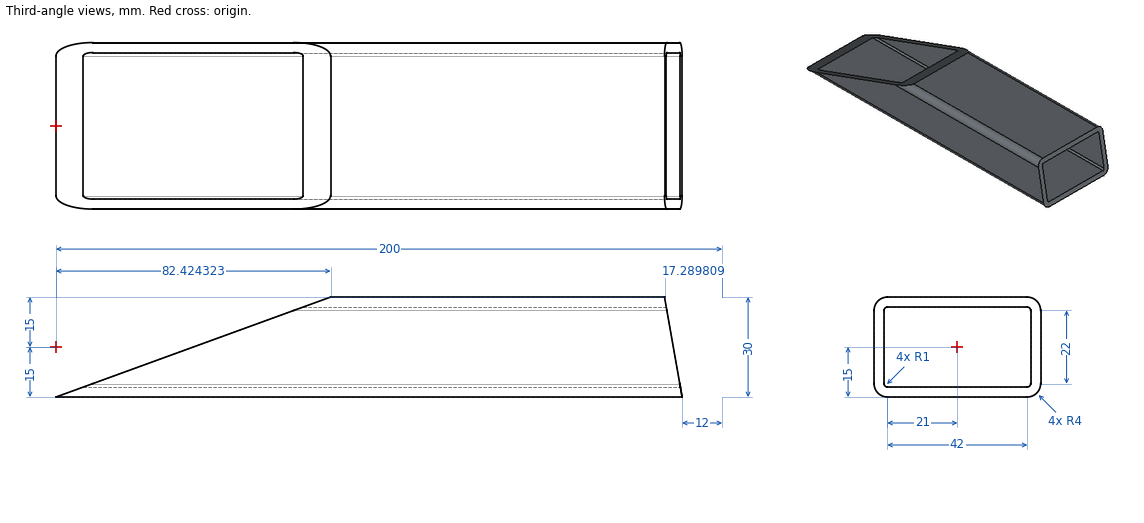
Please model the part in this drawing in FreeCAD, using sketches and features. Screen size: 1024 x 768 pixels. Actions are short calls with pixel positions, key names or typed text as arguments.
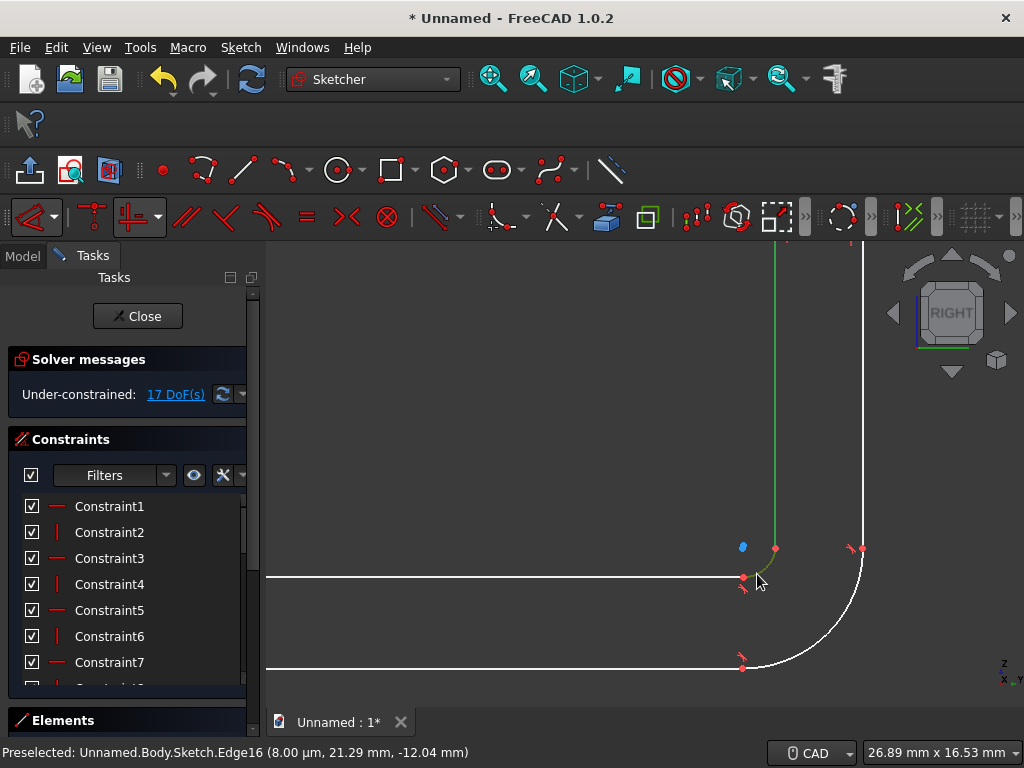
click(268, 218)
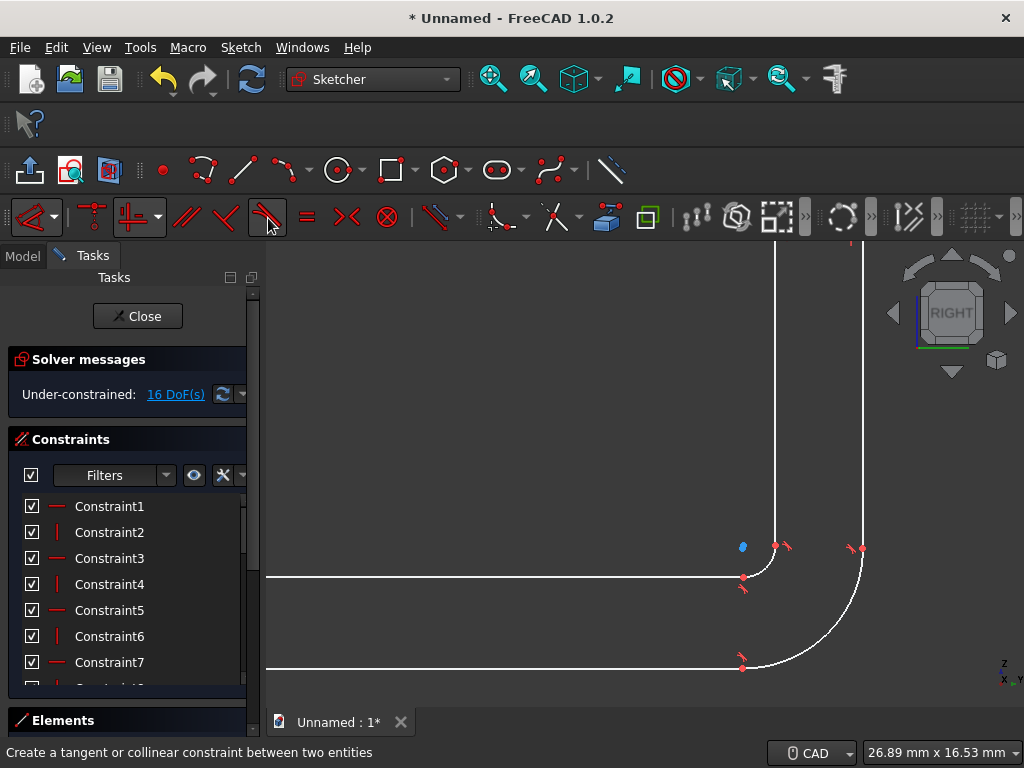
scroll(759, 576, down, 6)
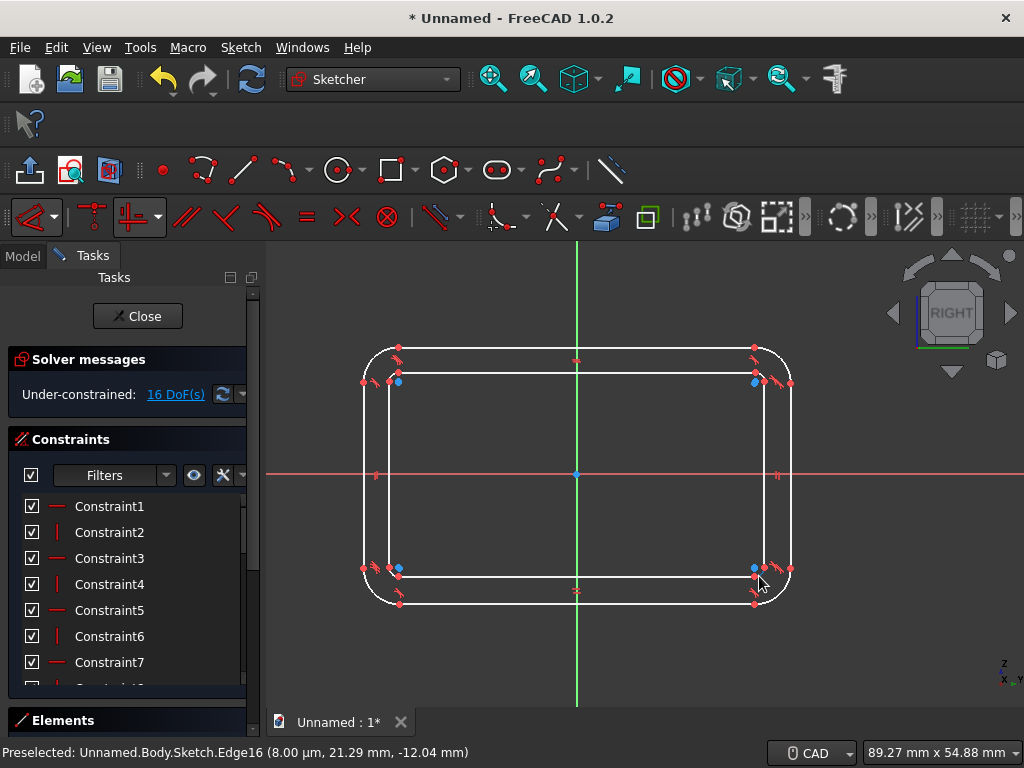
click(368, 585)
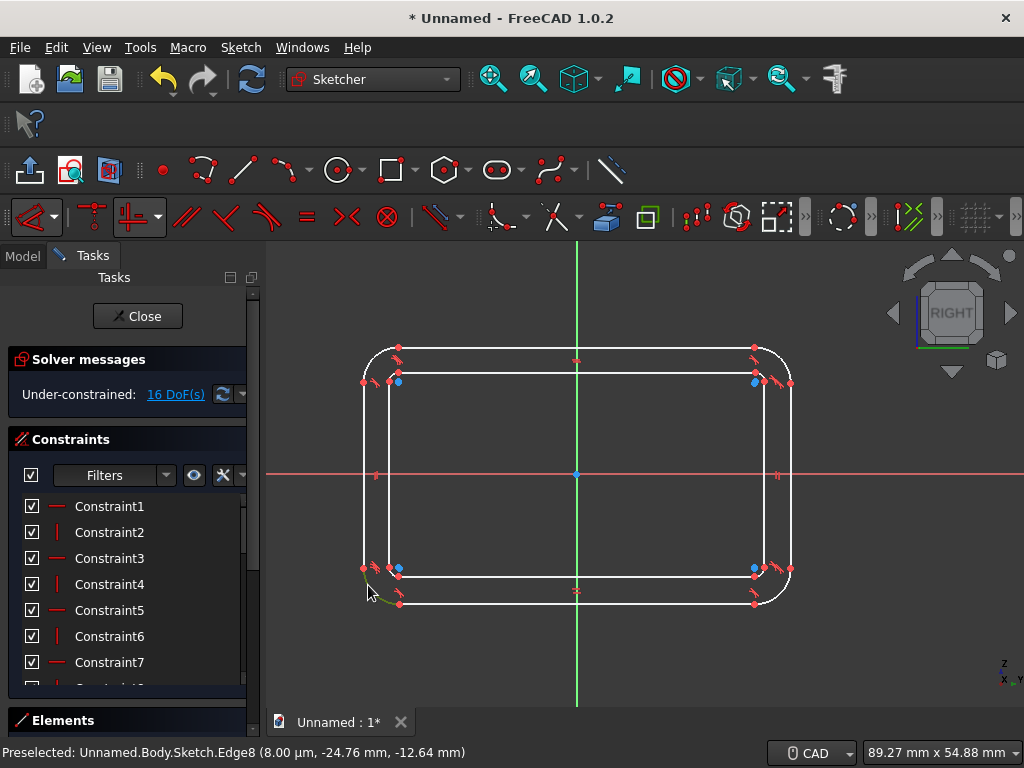
scroll(392, 574, up, 4)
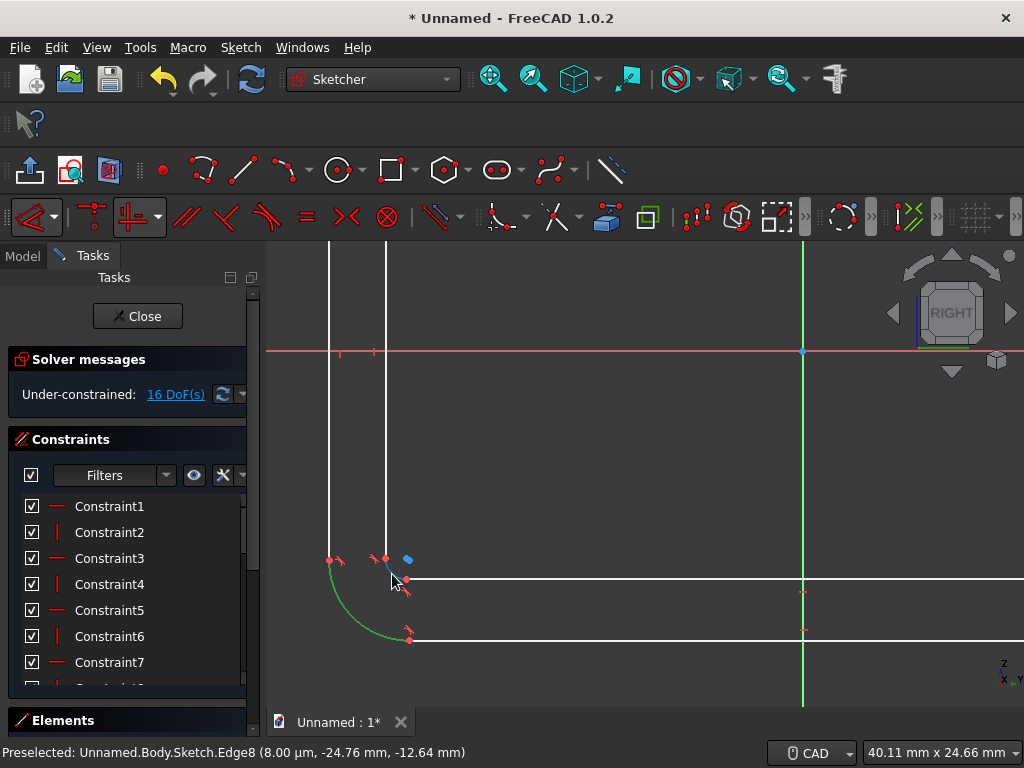
click(392, 573)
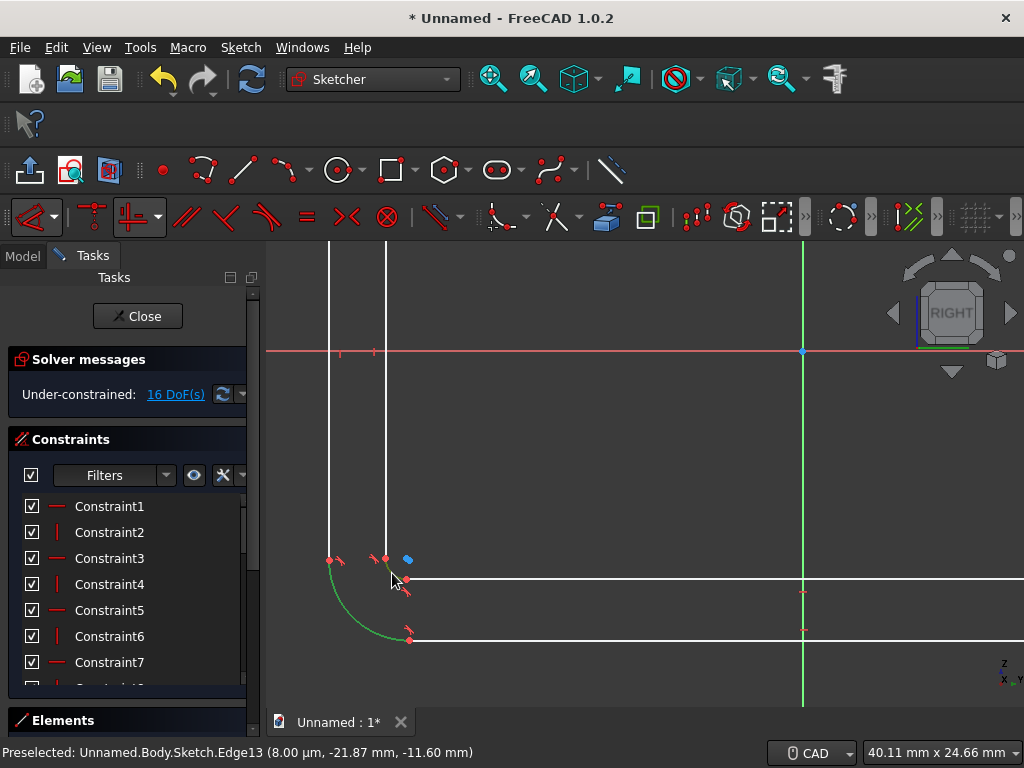
click(92, 218)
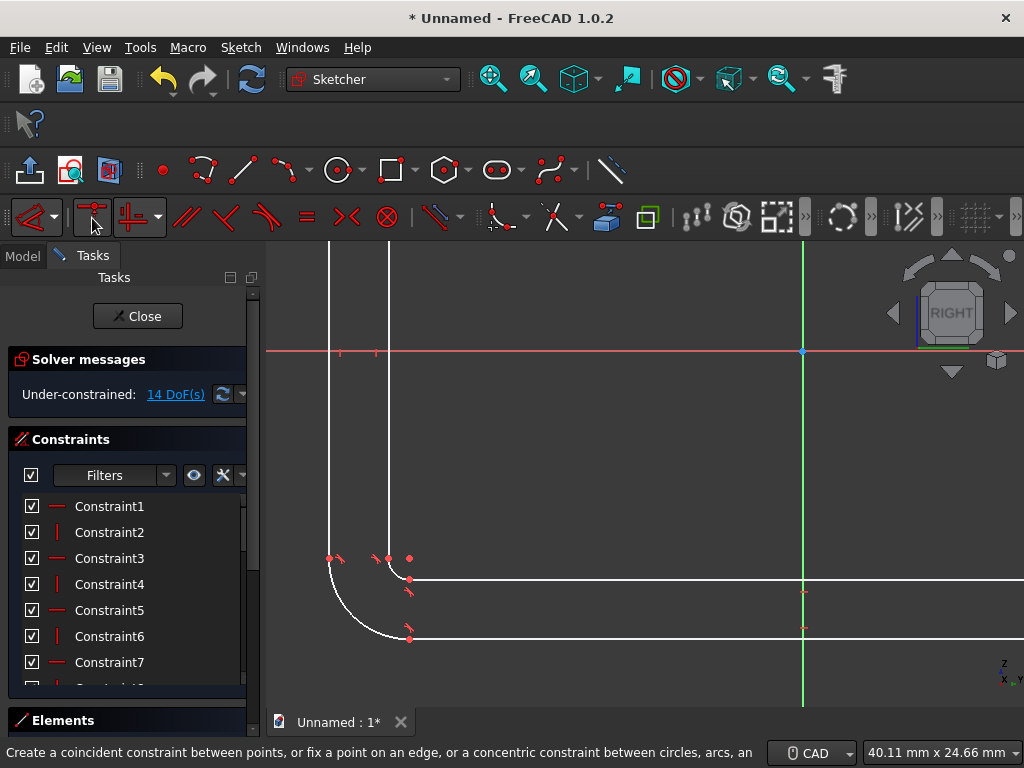
scroll(392, 574, down, 4)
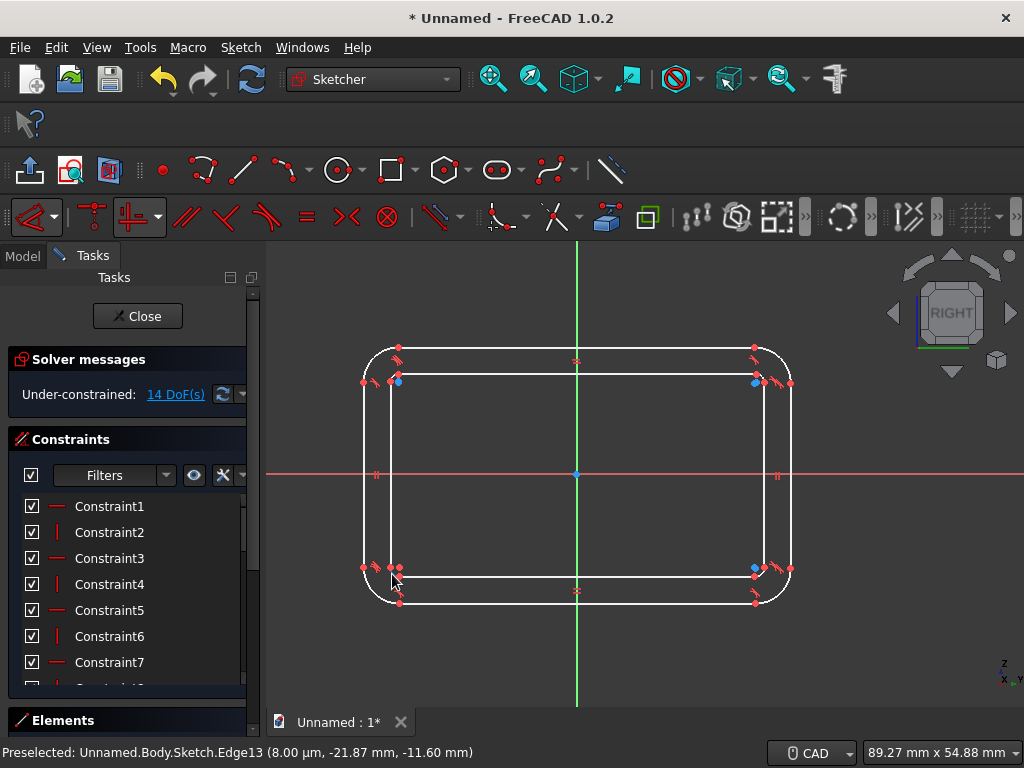
click(383, 351)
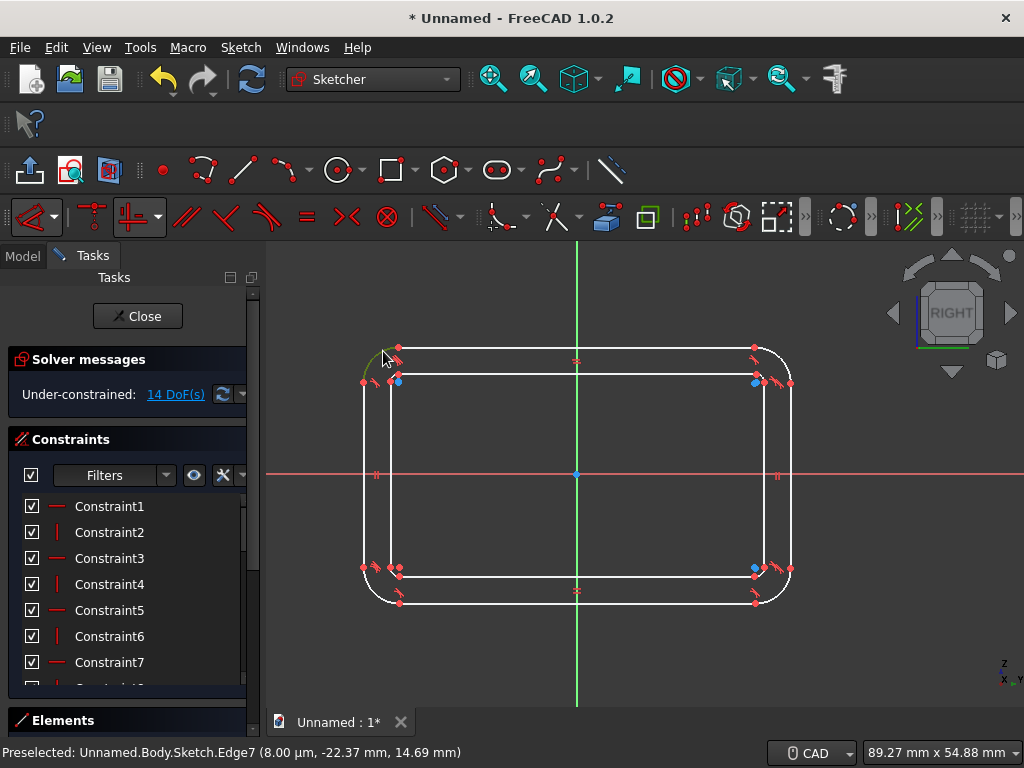
scroll(393, 376, up, 5)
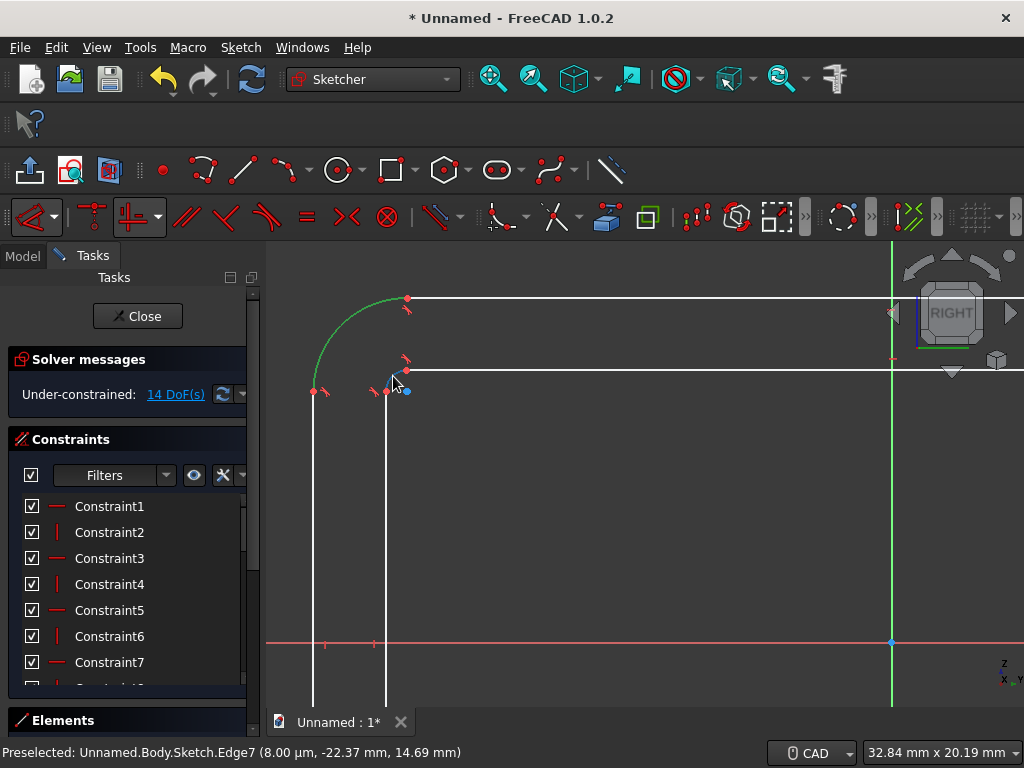
click(392, 376)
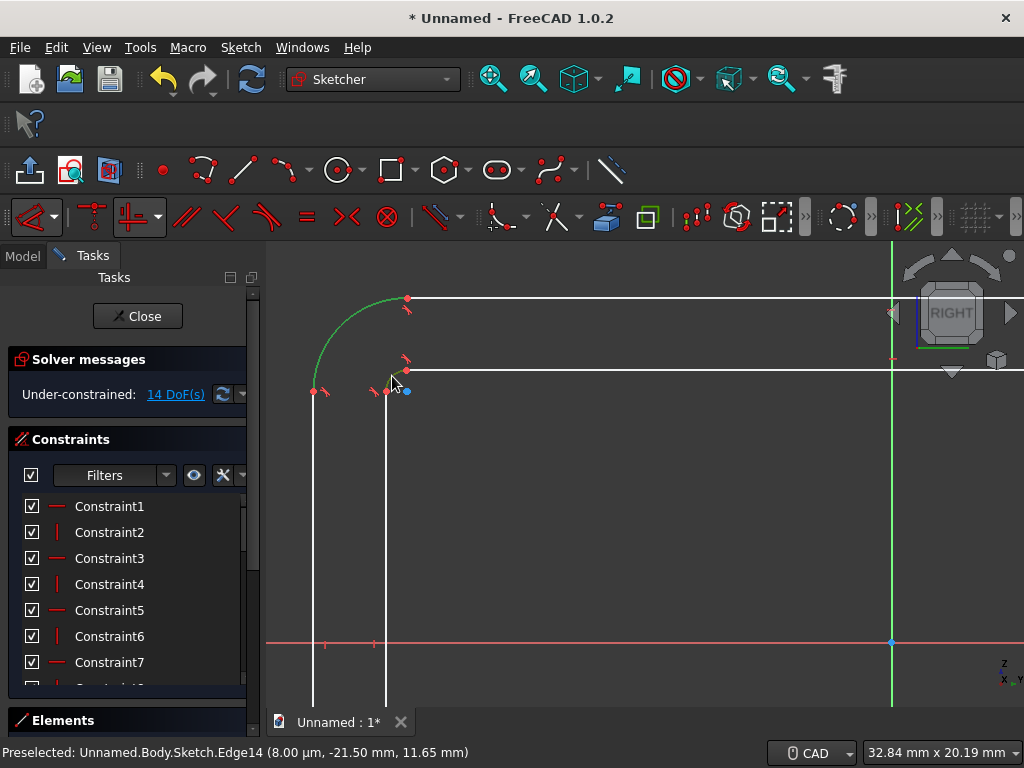
click(92, 218)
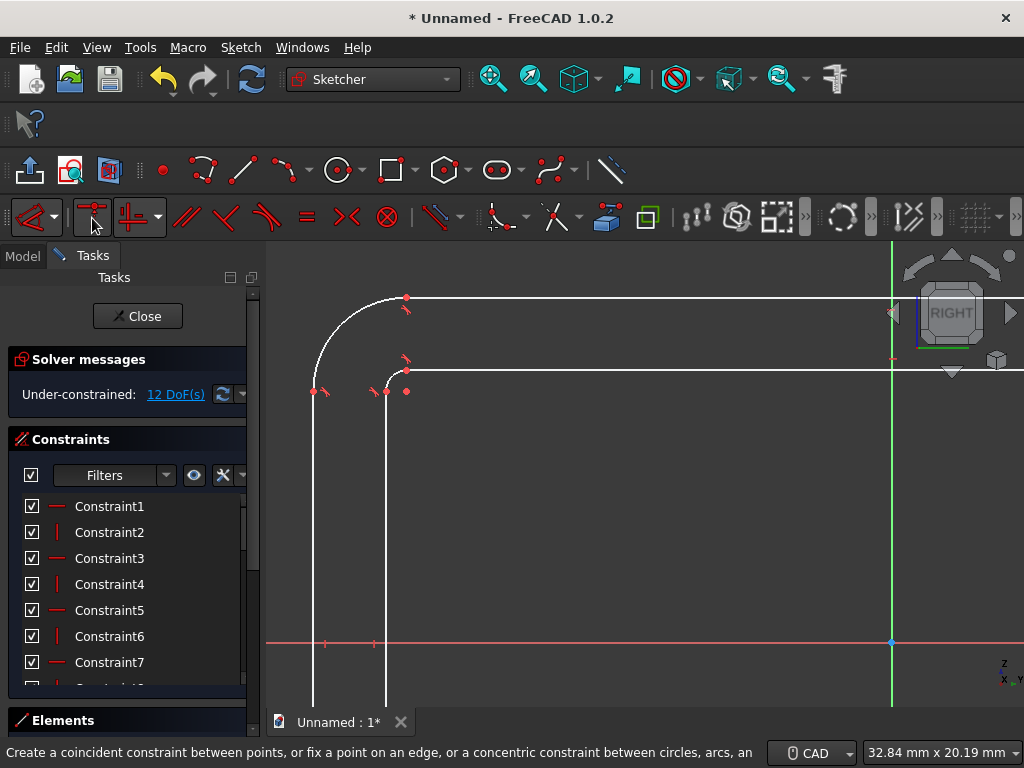
scroll(393, 376, down, 5)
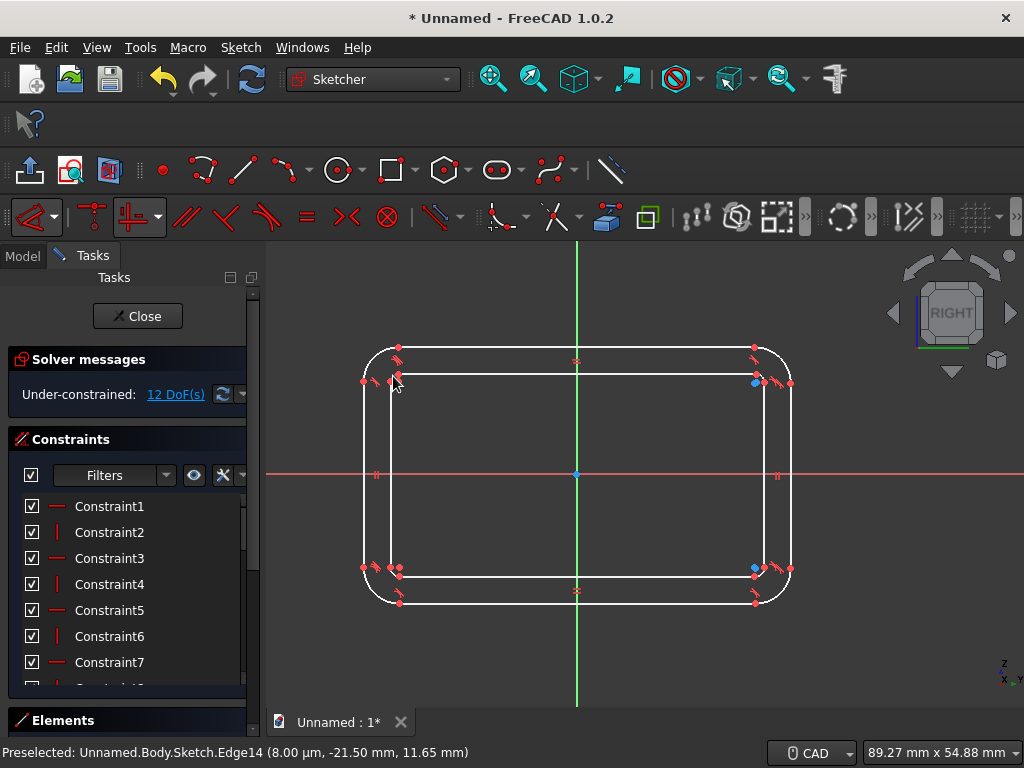
click(787, 367)